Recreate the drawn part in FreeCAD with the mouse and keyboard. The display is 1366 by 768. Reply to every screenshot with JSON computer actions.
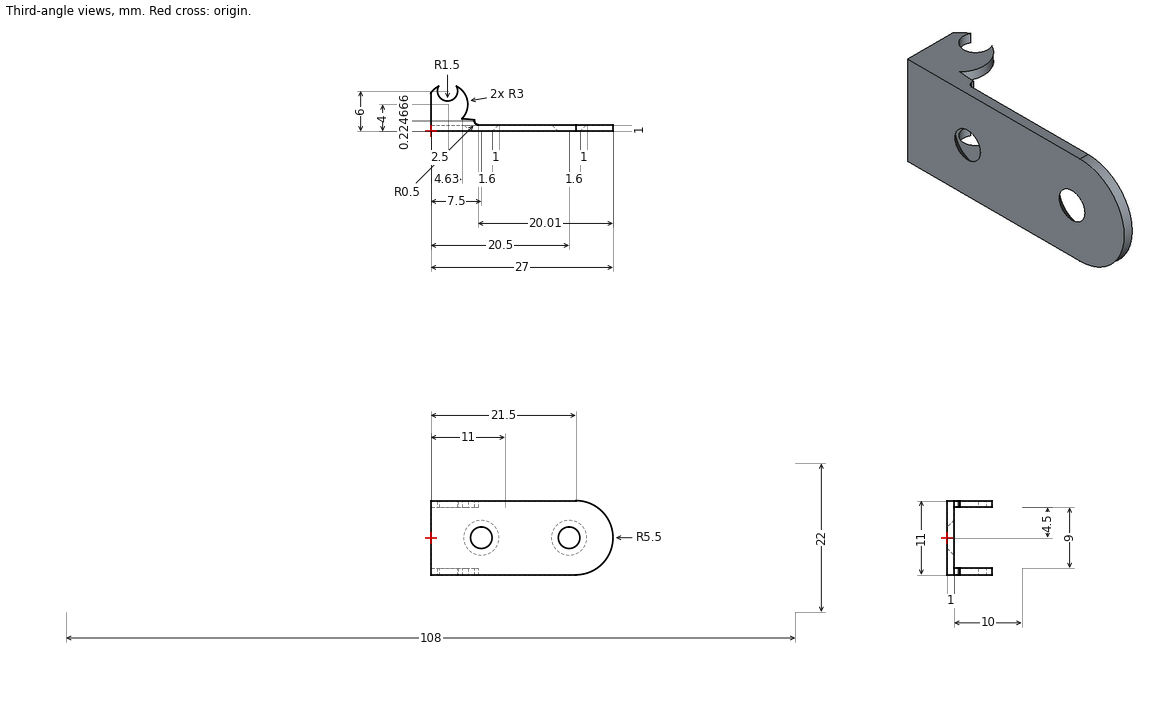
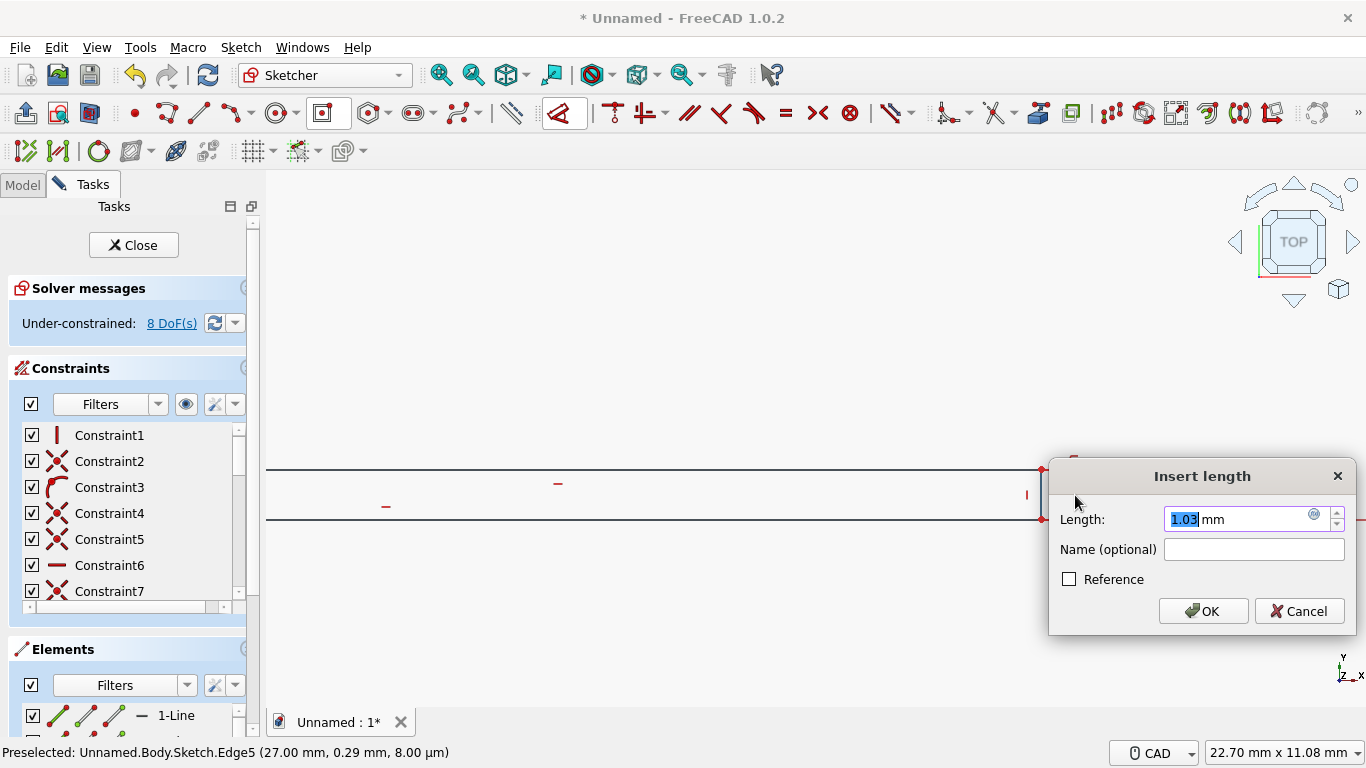
{"action": "type", "text": "1"}
{"action": "key", "text": "Return"}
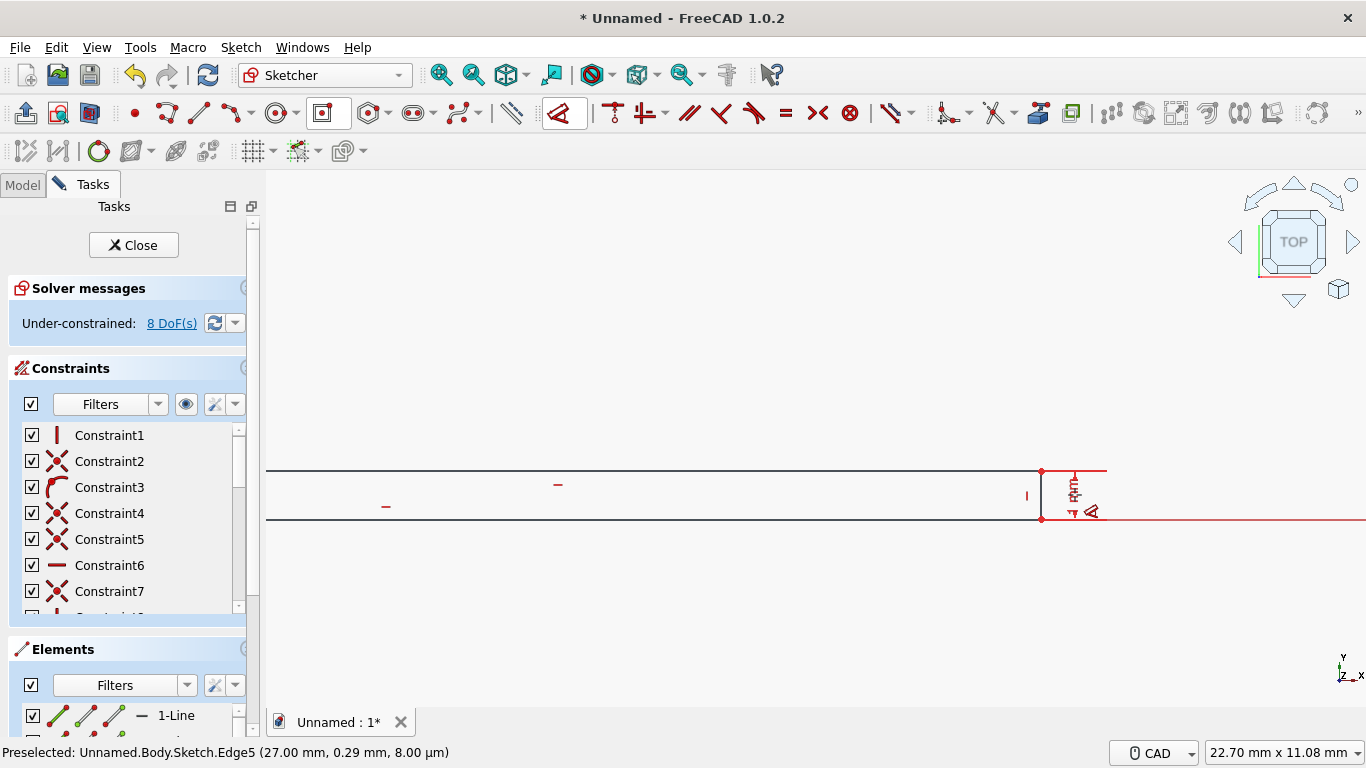
{"action": "left_click", "coordinate": [648, 520]}
{"action": "left_click", "coordinate": [668, 554]}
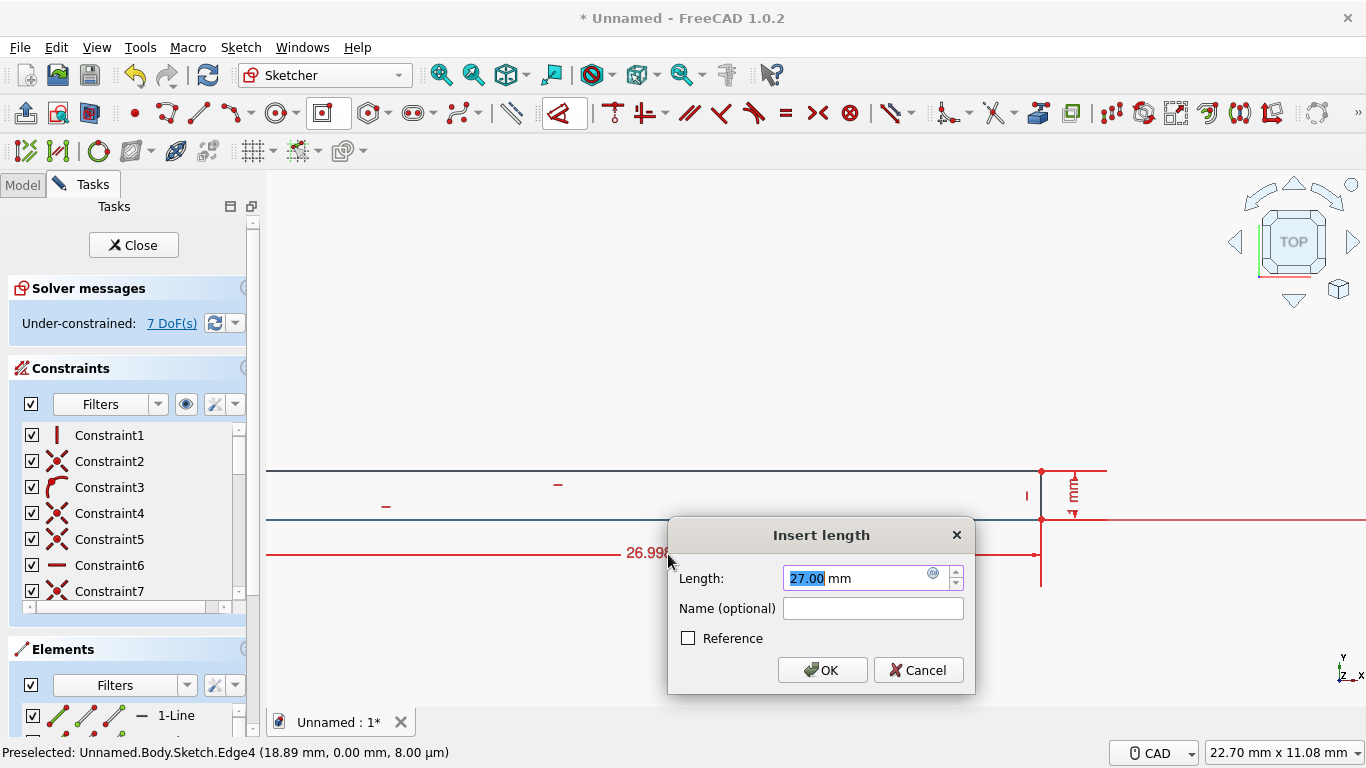
{"action": "type", "text": "27"}
{"action": "key", "text": "Return"}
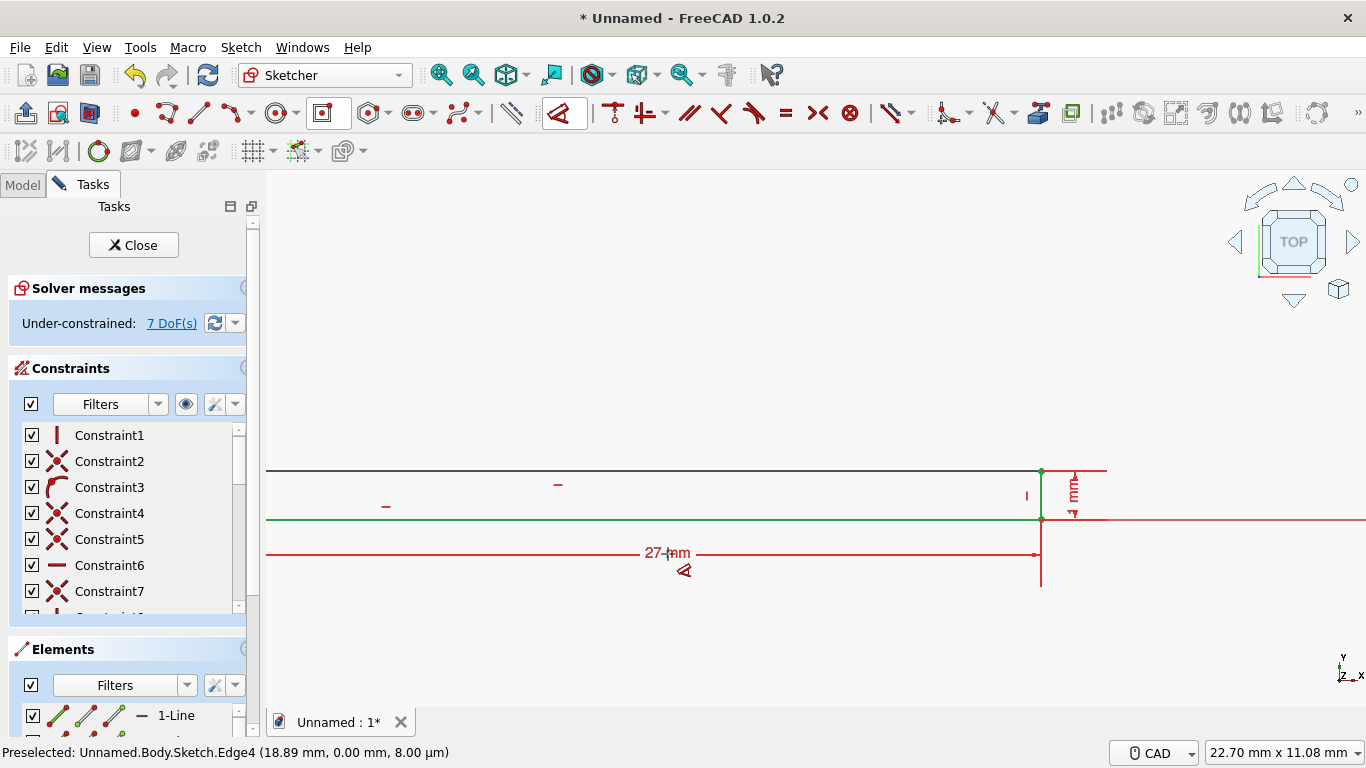
{"action": "scroll", "coordinate": [1042, 504], "scroll_direction": "down", "scroll_amount": 4}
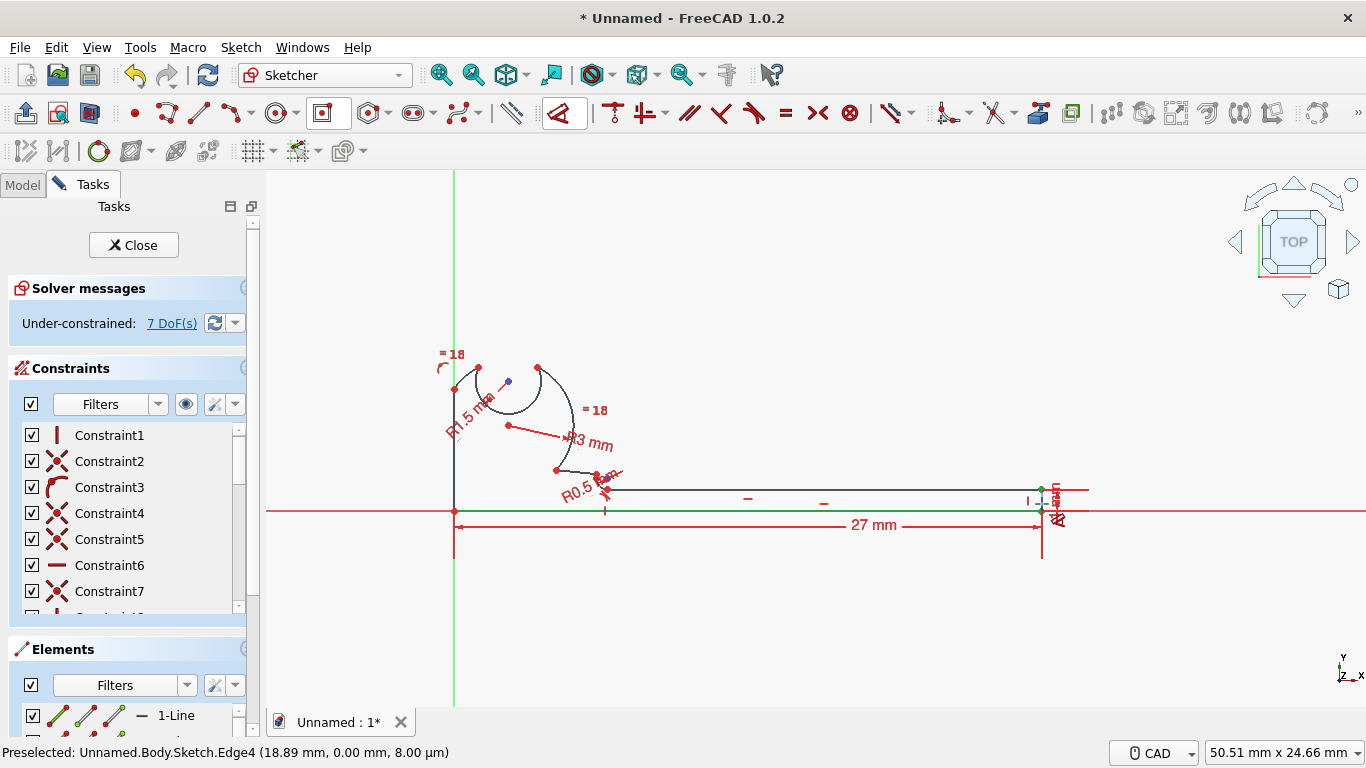
{"action": "left_click", "coordinate": [508, 426]}
{"action": "left_click", "coordinate": [420, 469]}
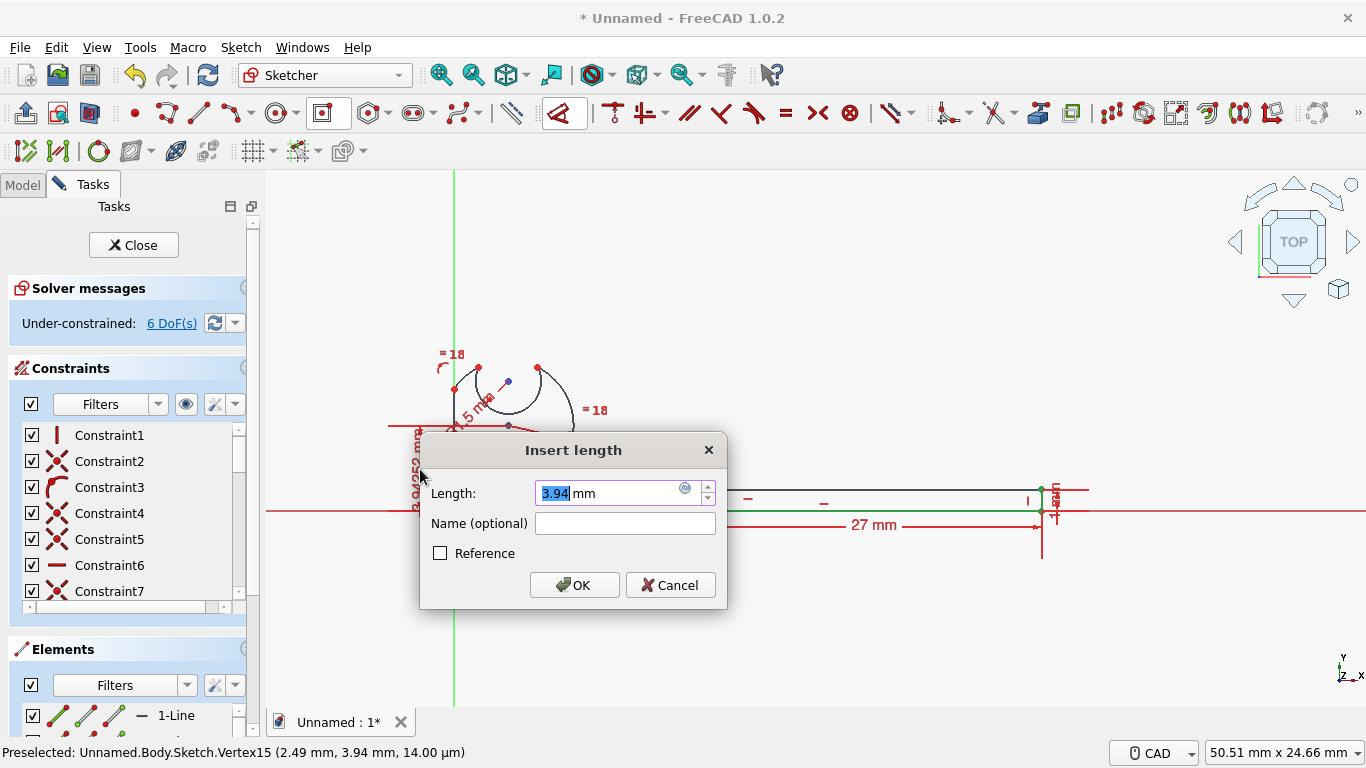
{"action": "type", "text": "4"}
{"action": "key", "text": "Return"}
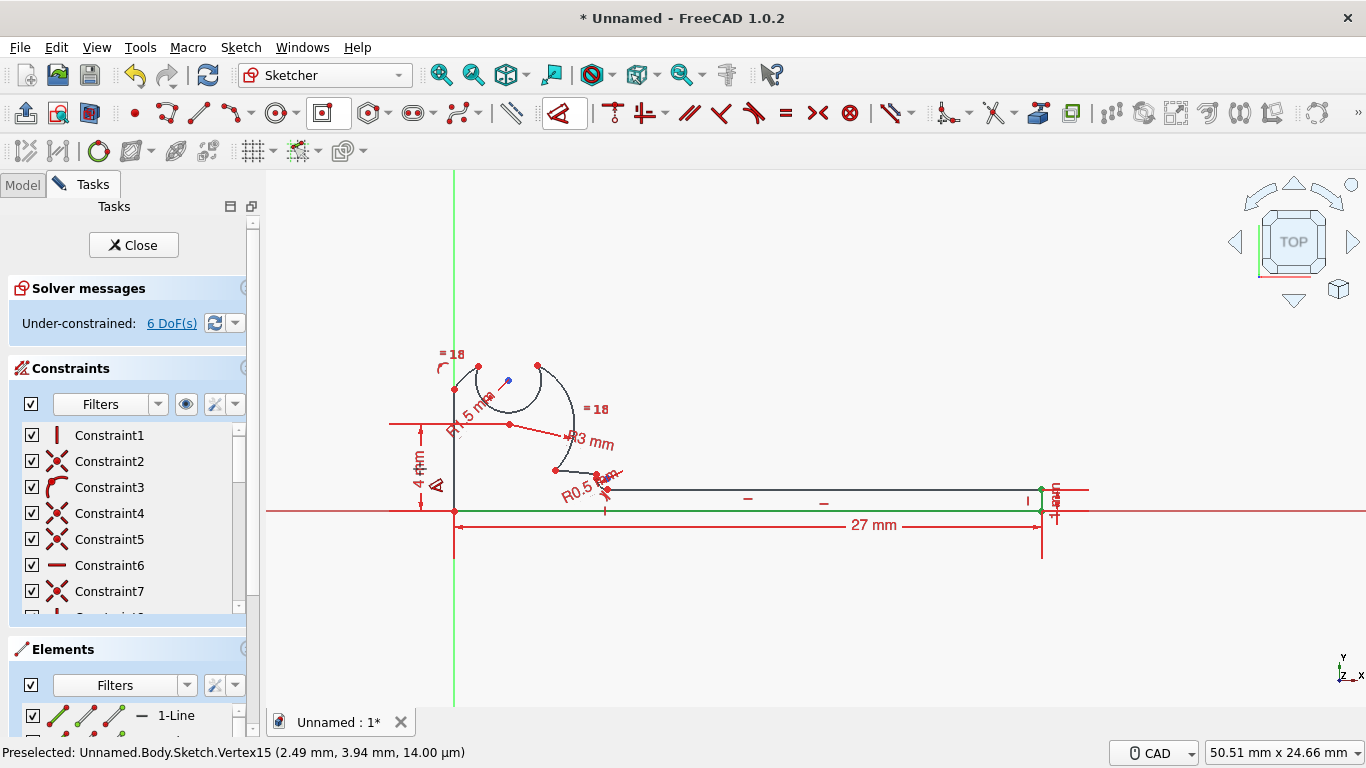
{"action": "left_click", "coordinate": [509, 380]}
{"action": "left_click", "coordinate": [420, 446]}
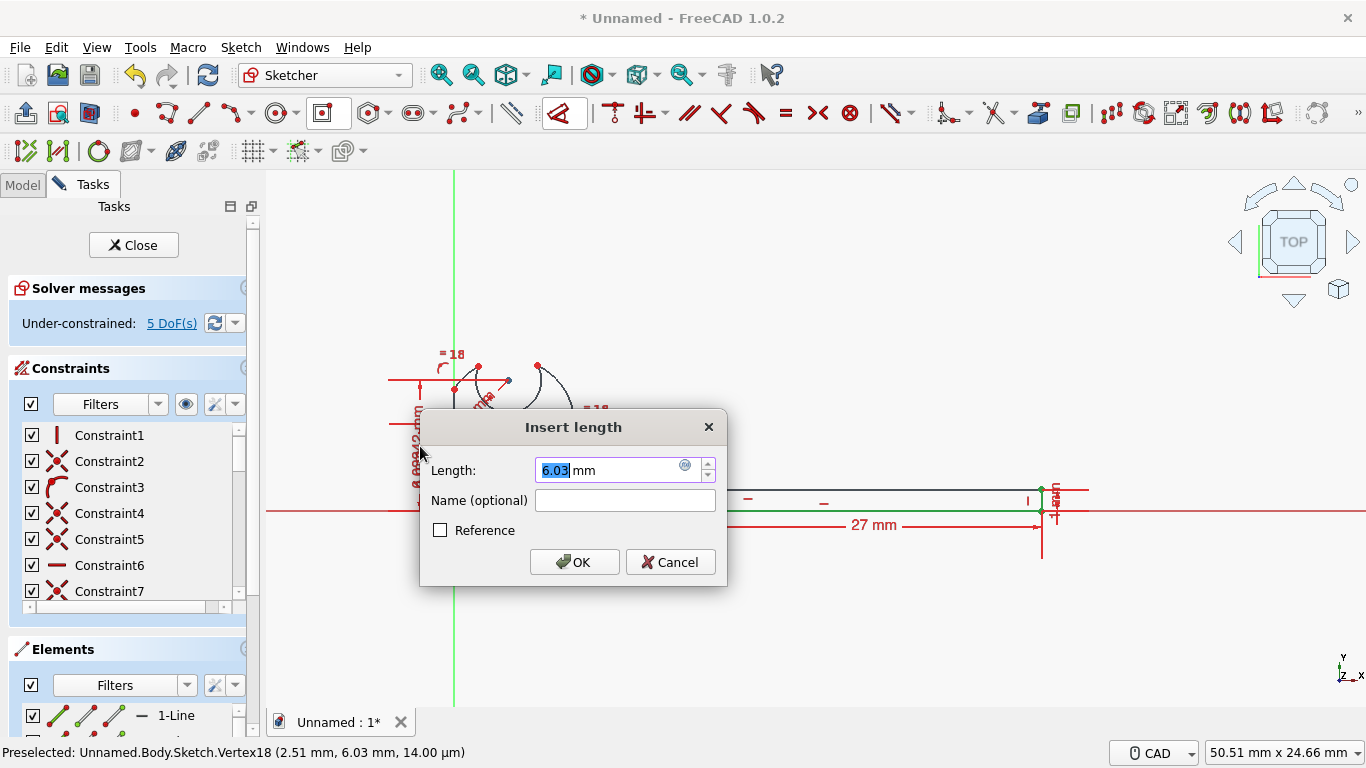
{"action": "type", "text": "6"}
{"action": "key", "text": "Return"}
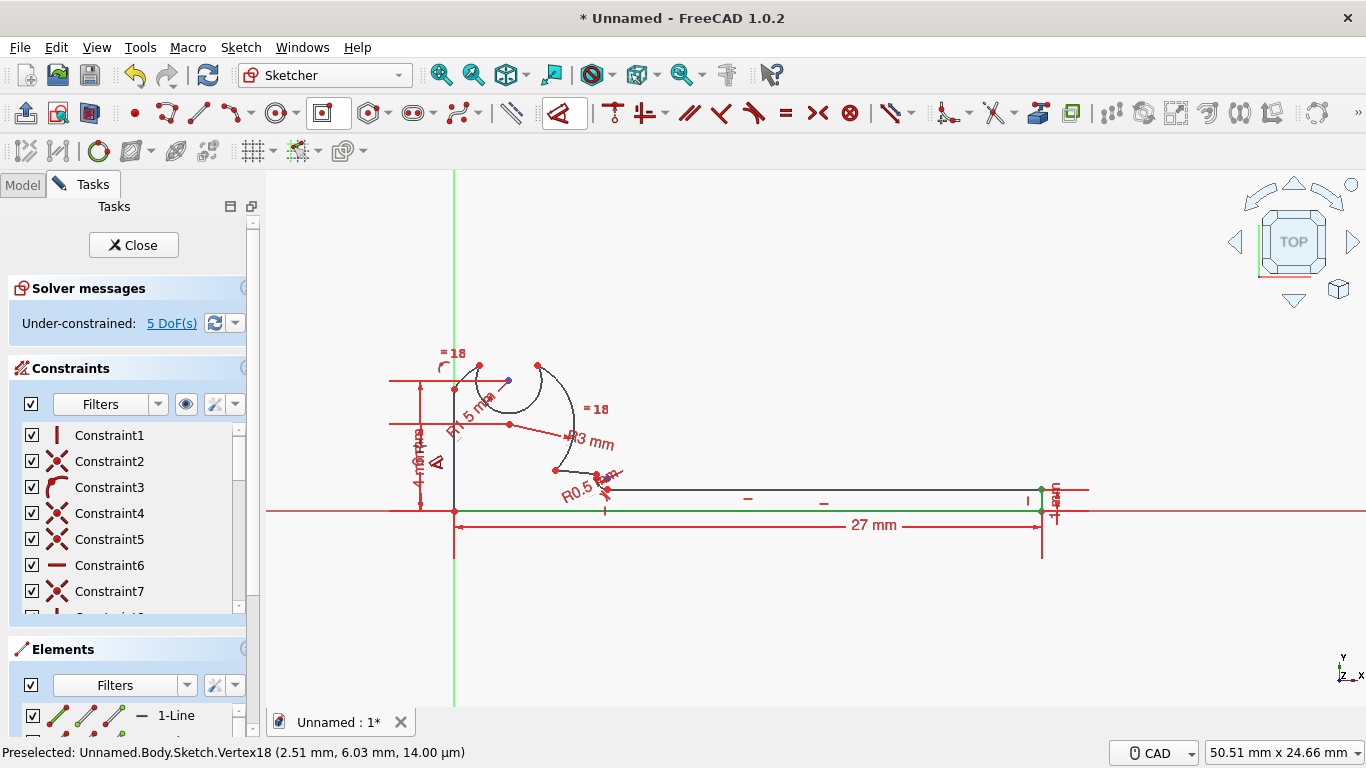
{"action": "left_click", "coordinate": [509, 424]}
{"action": "left_click", "coordinate": [482, 545]}